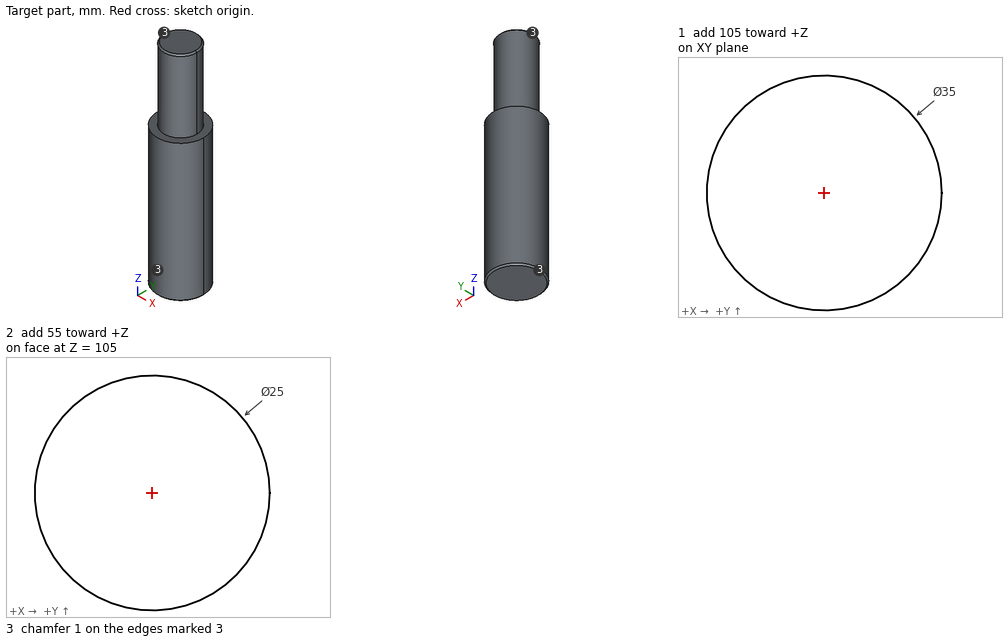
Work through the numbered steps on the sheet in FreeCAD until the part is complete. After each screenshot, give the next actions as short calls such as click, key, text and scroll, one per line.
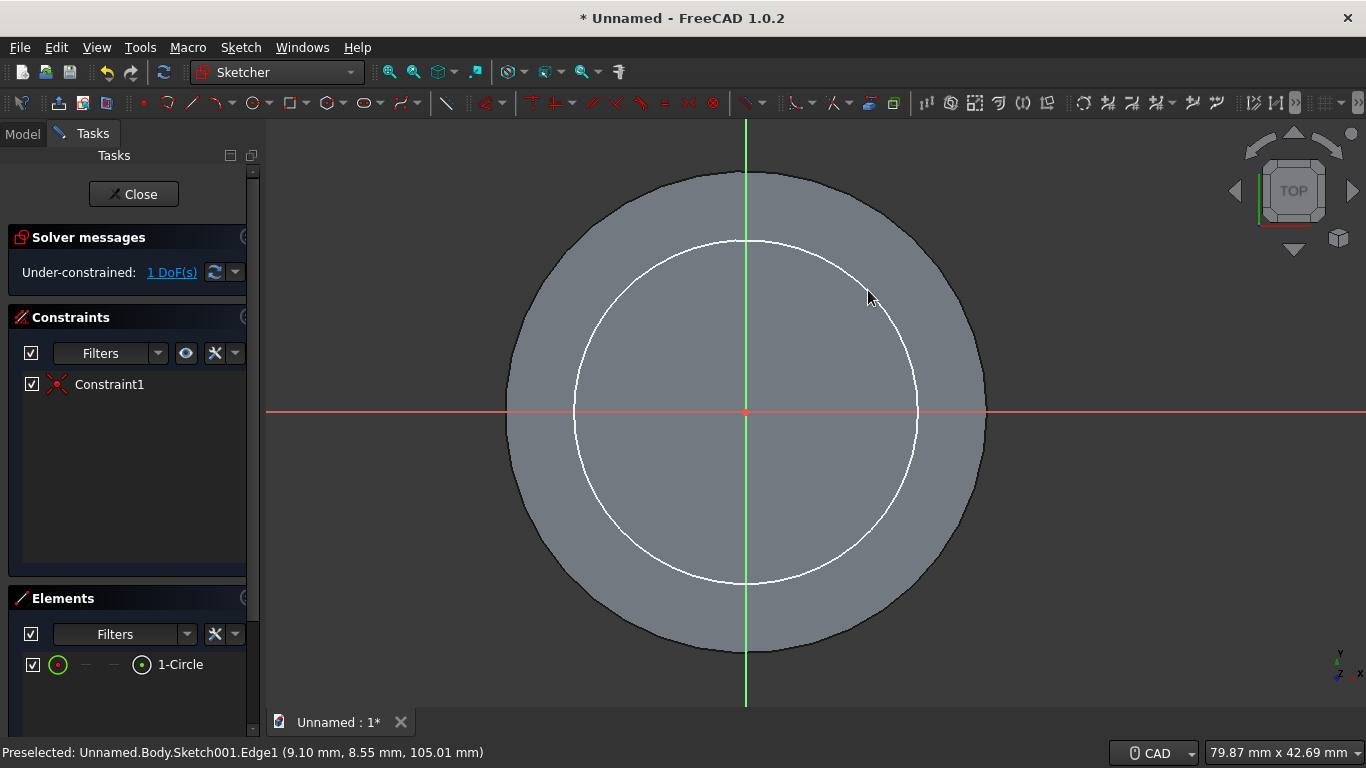
click(486, 104)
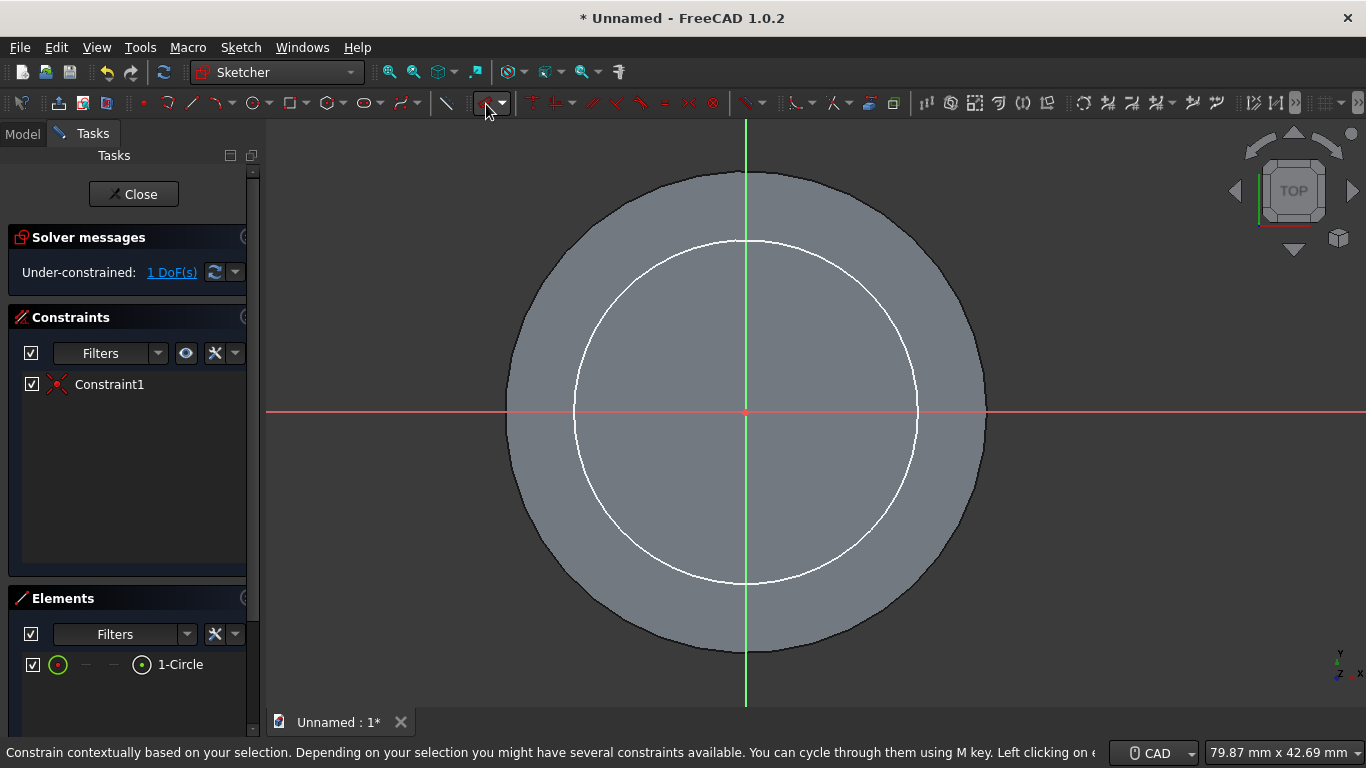
click(867, 290)
click(890, 267)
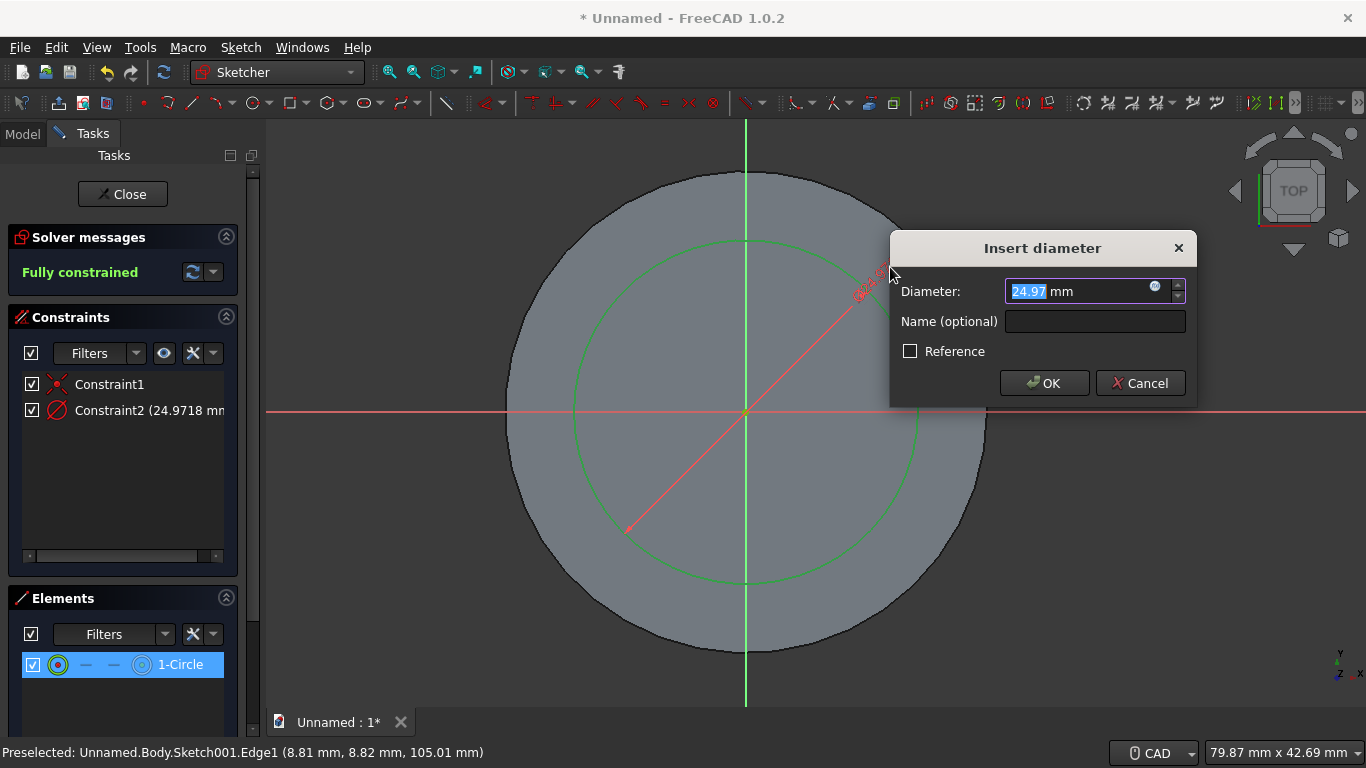
text(25)
key(Return)
key(Escape)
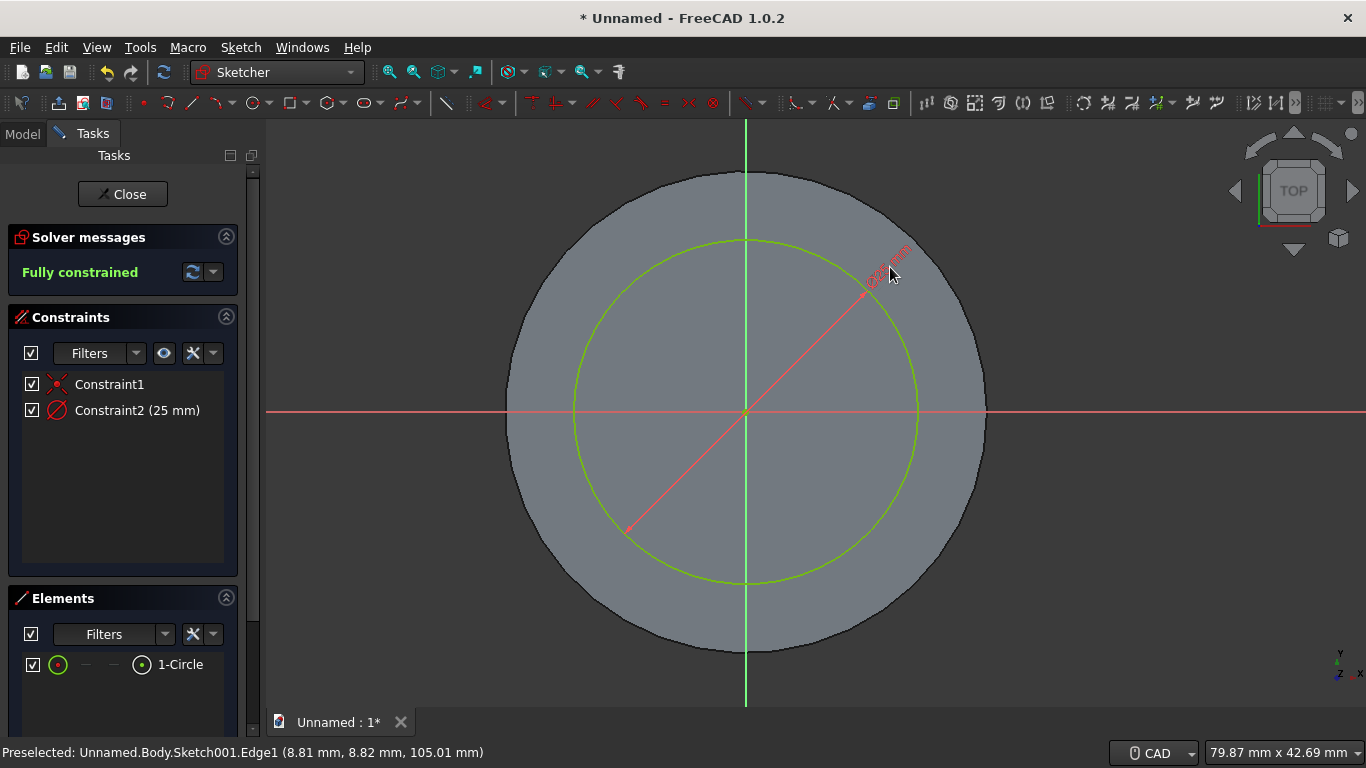
click(123, 194)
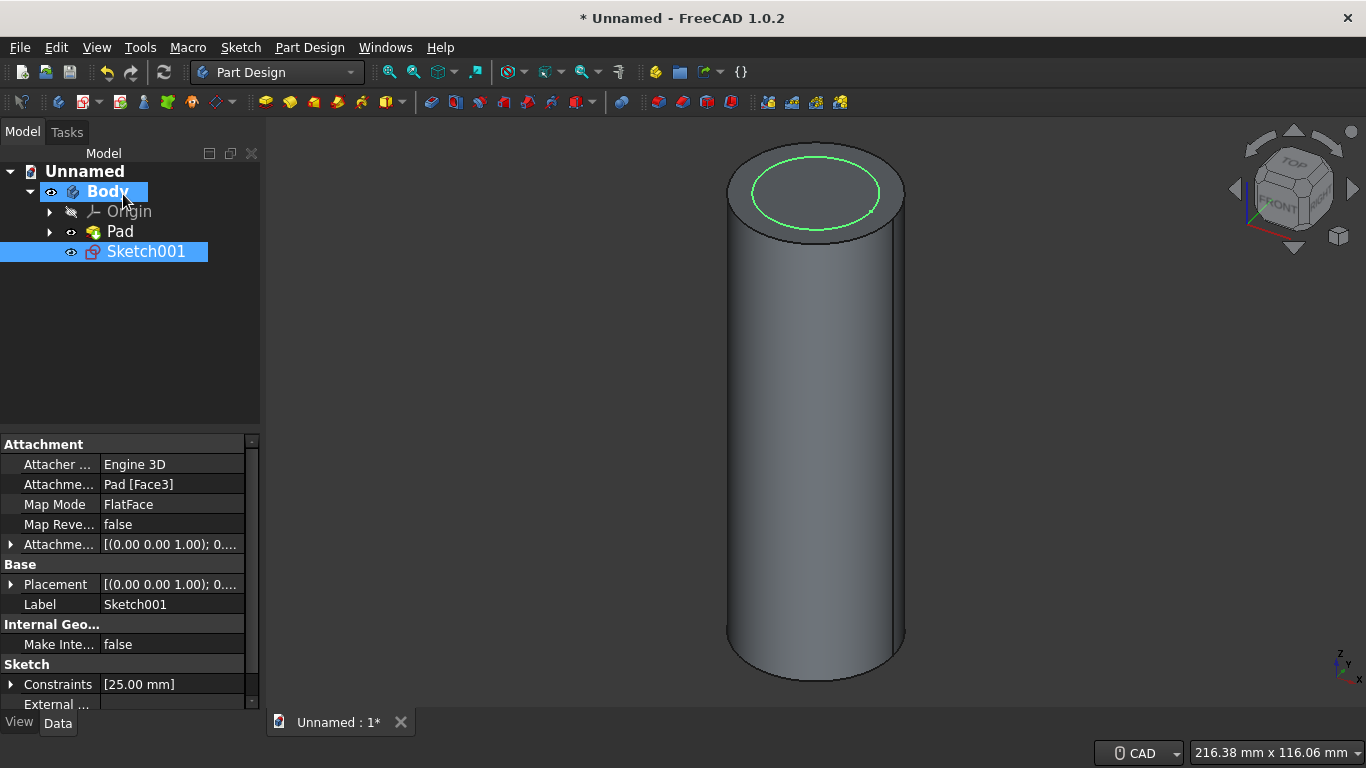
click(266, 102)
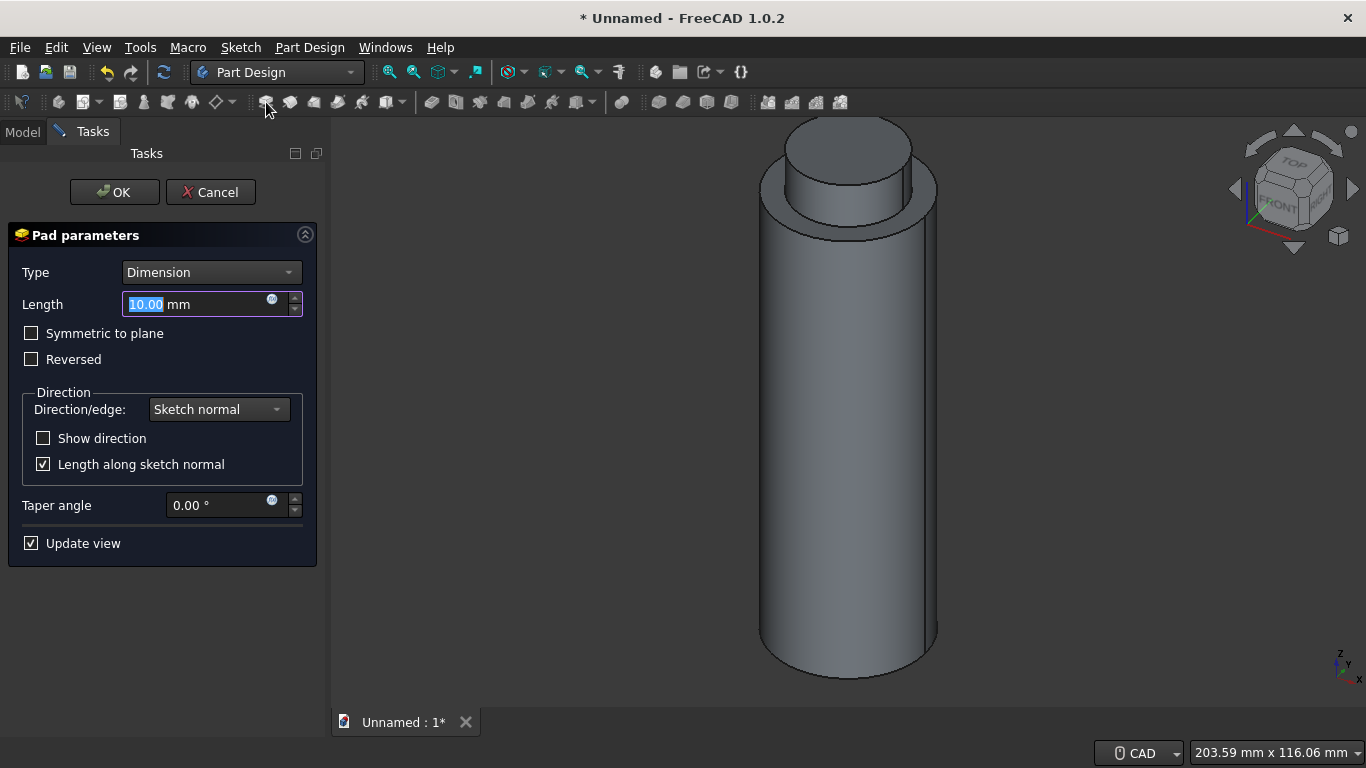
text(55)
key(Tab)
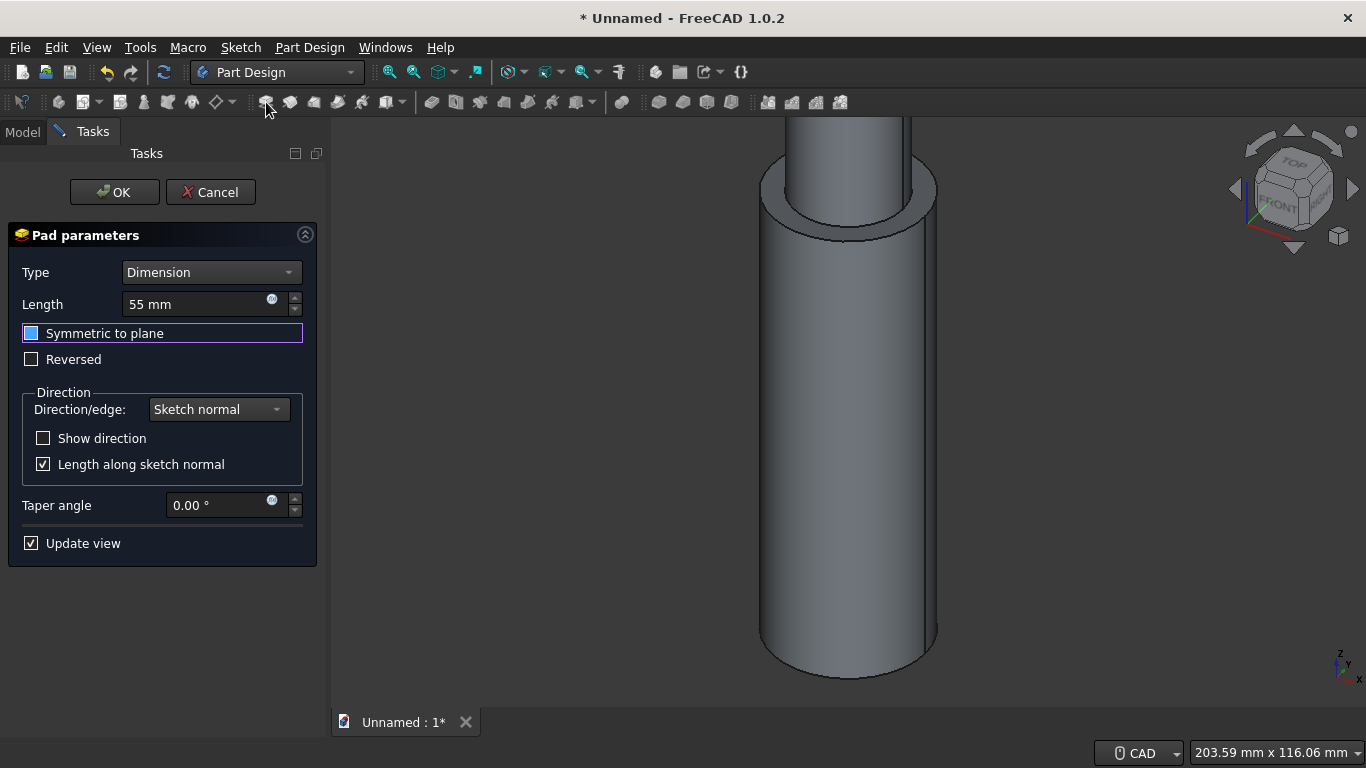
click(115, 192)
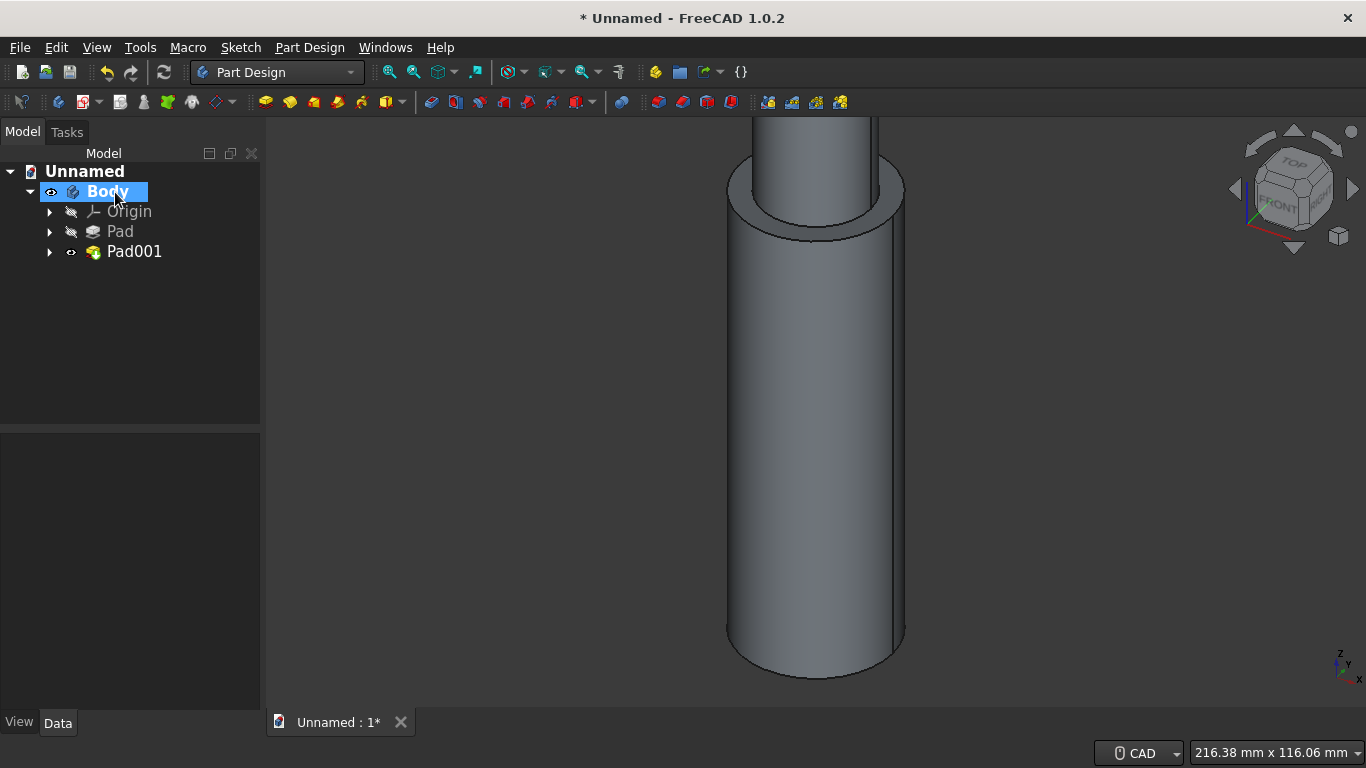
click(390, 72)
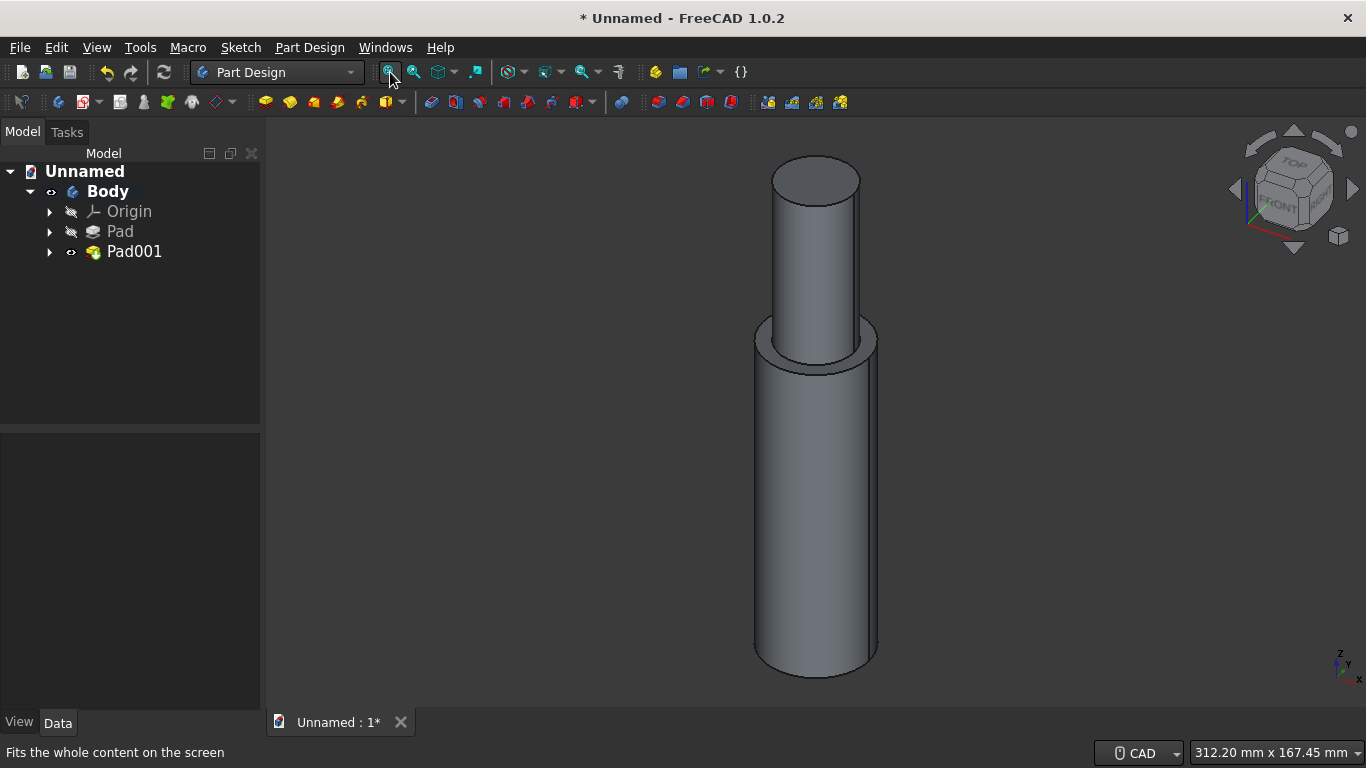
click(770, 666)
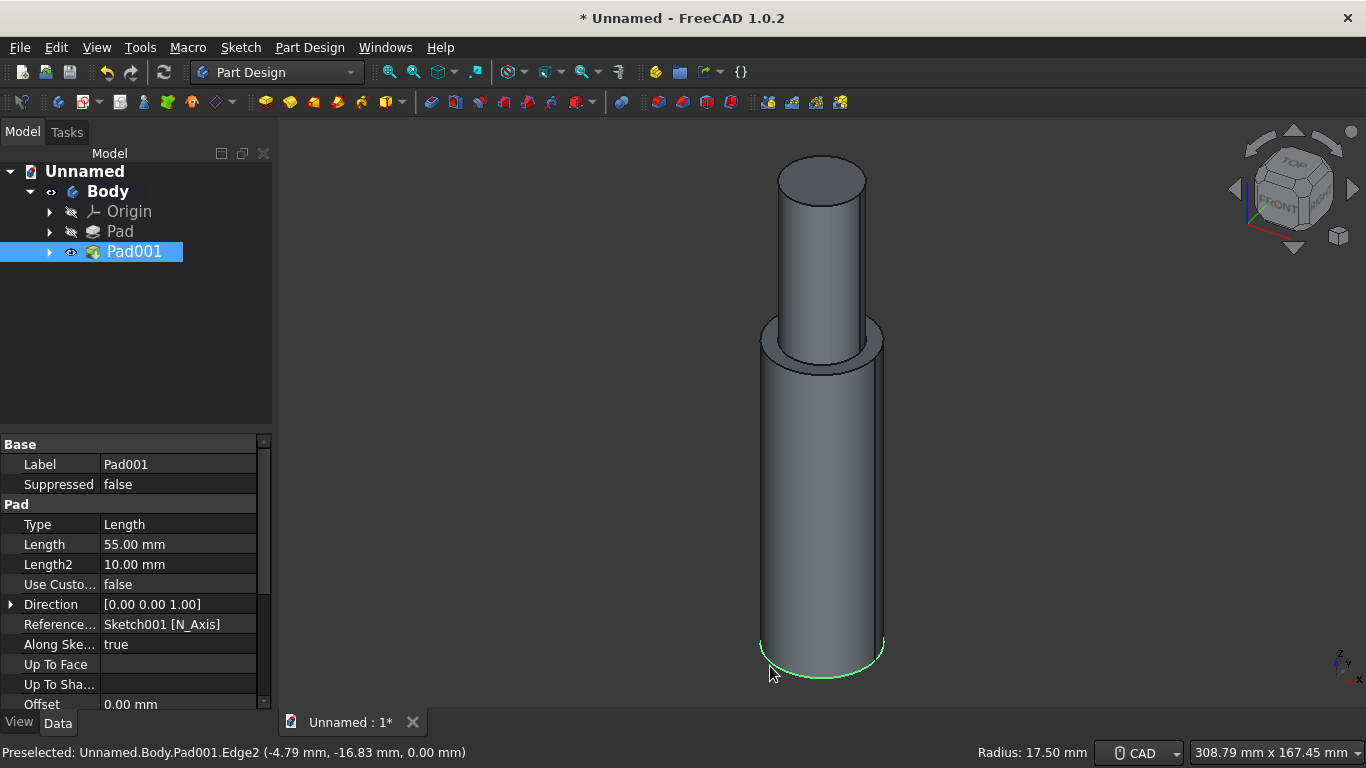
click(778, 183, ctrl)